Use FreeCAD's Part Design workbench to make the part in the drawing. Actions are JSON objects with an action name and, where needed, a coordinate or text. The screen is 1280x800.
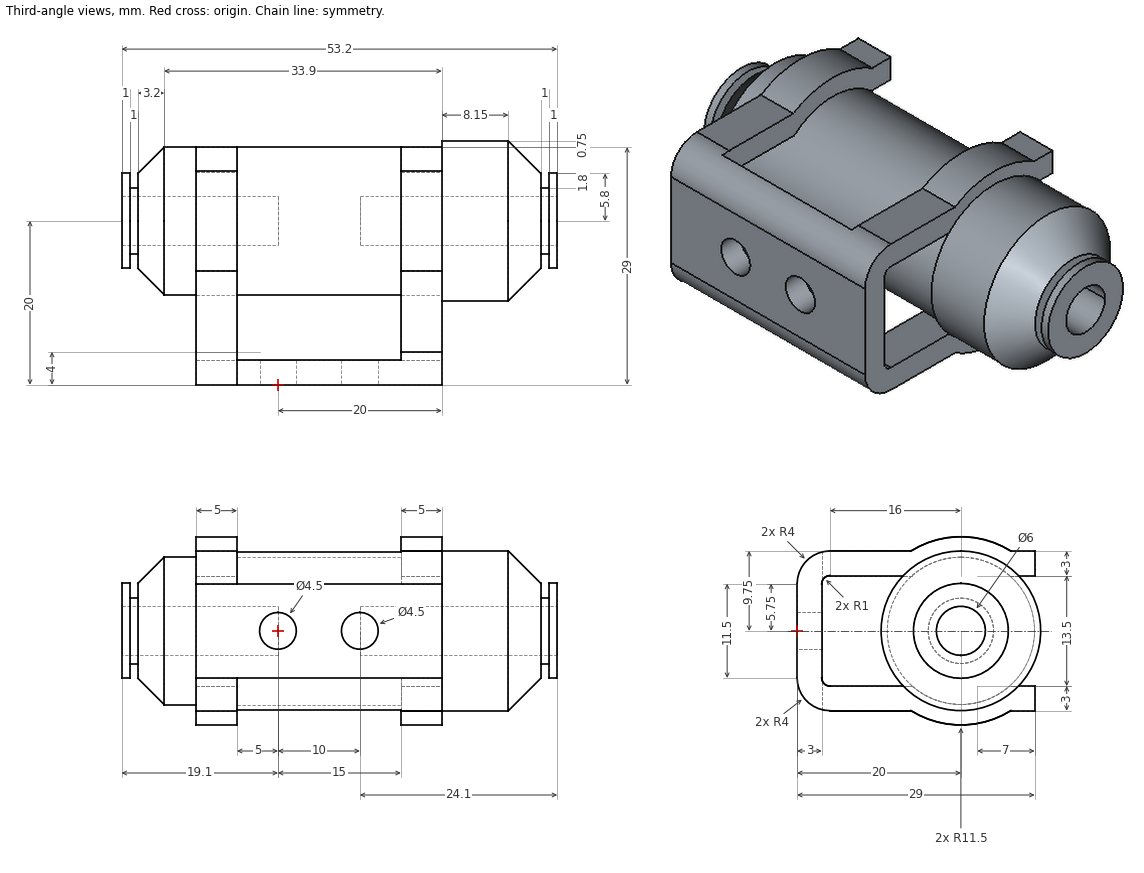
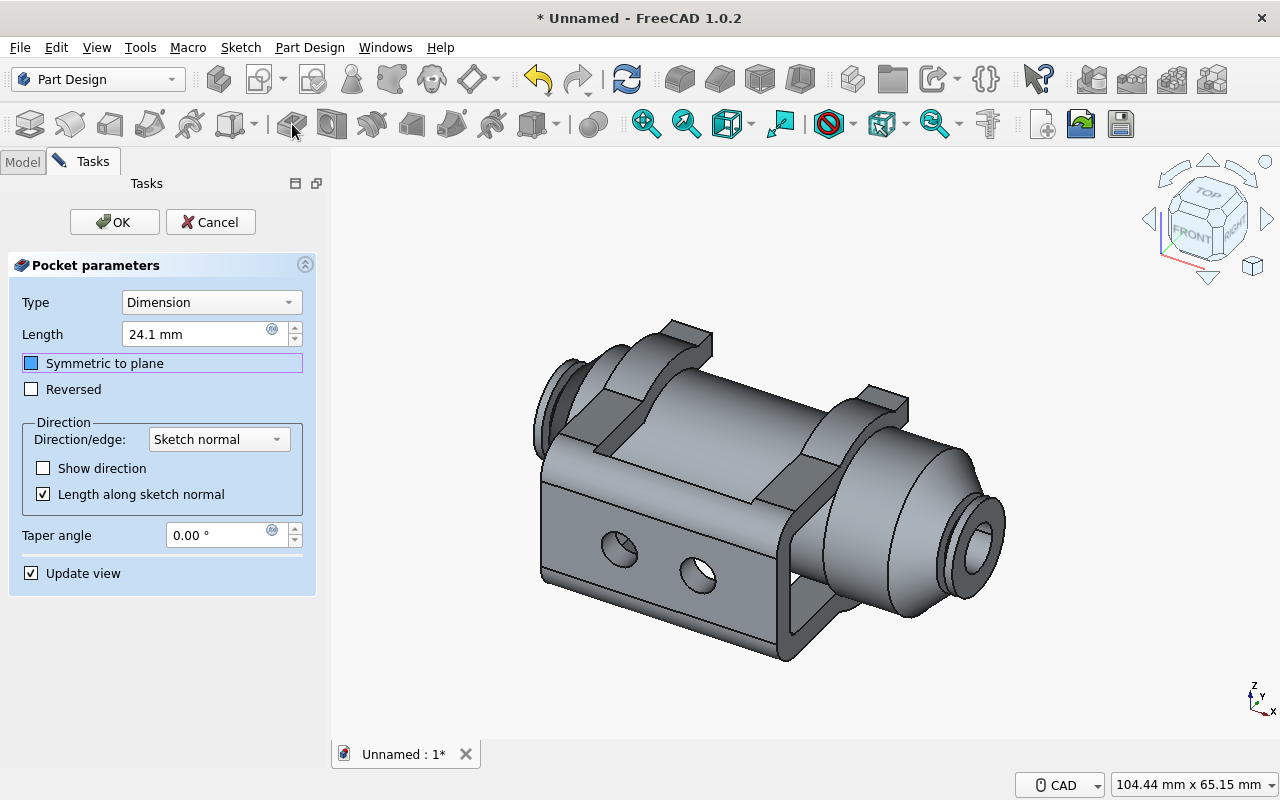
{"action": "left_click", "coordinate": [115, 222]}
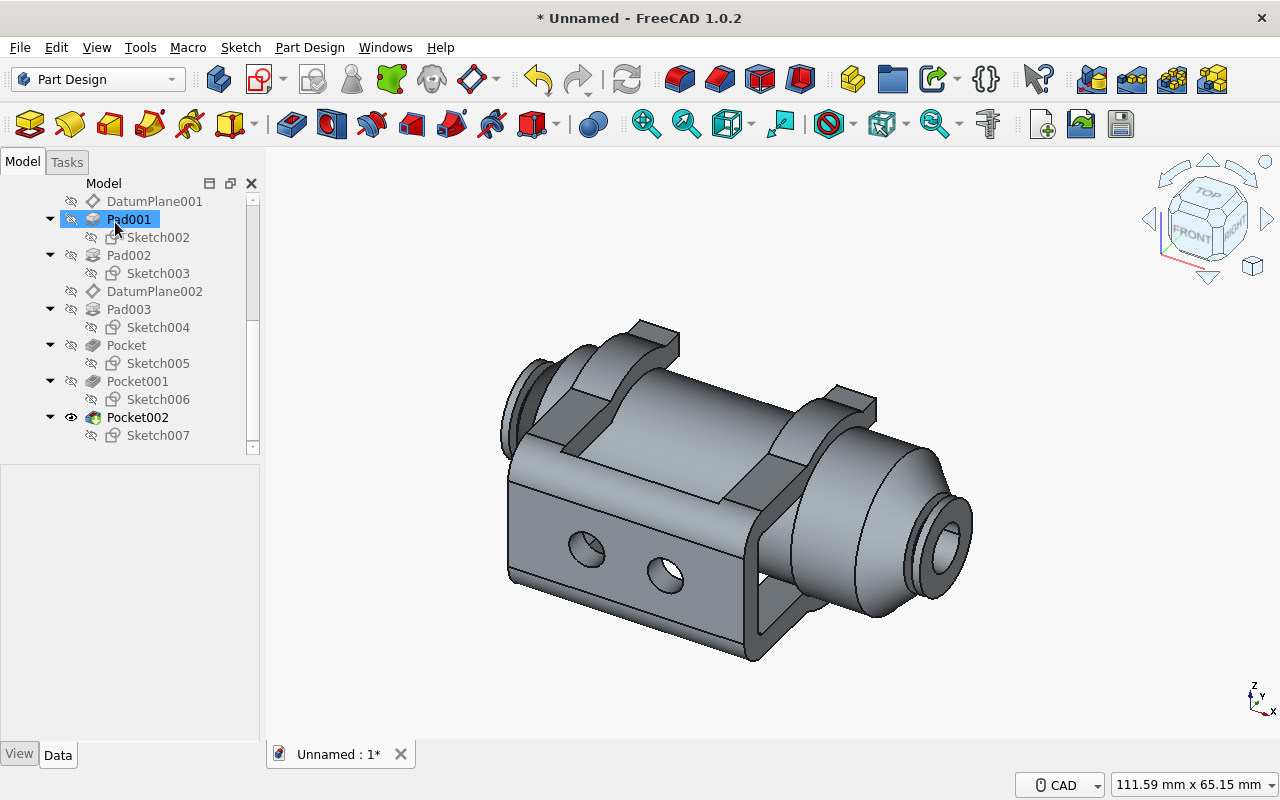
{"action": "left_click", "coordinate": [260, 80]}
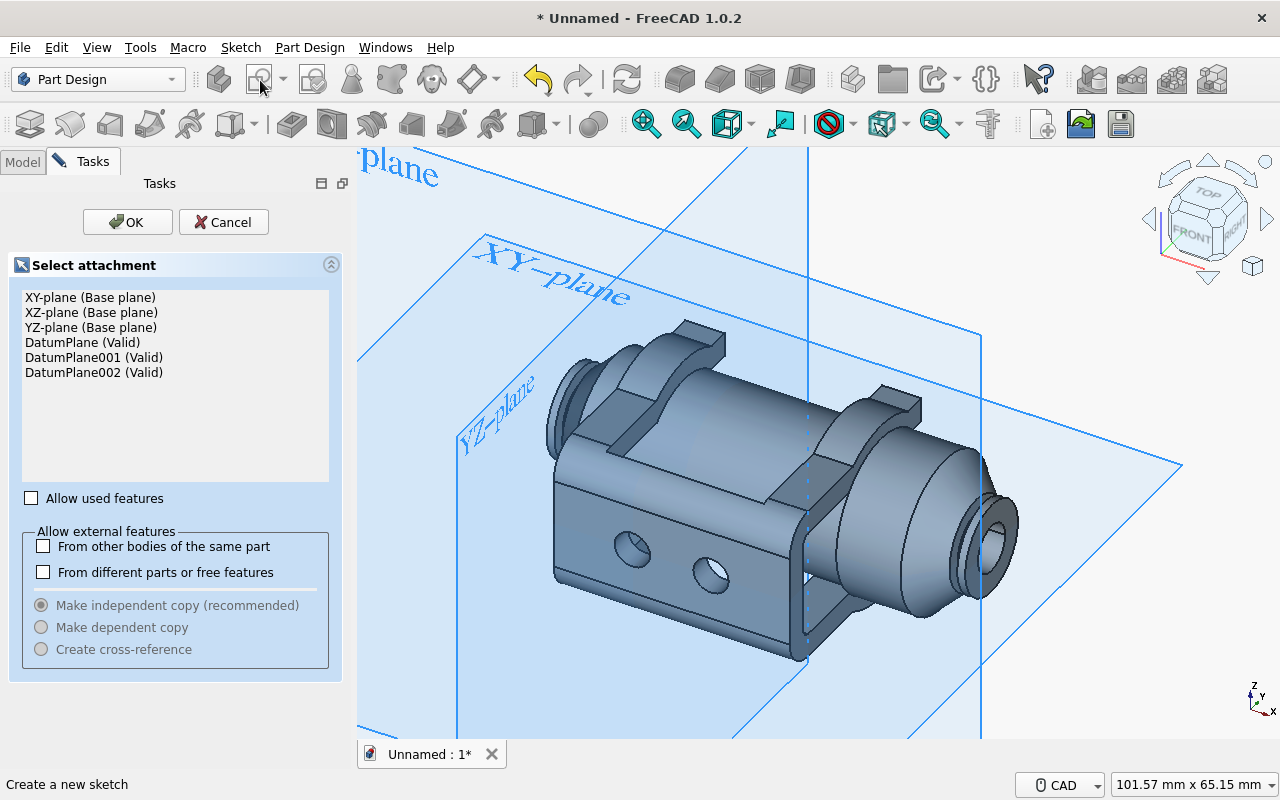
{"action": "left_click", "coordinate": [82, 328]}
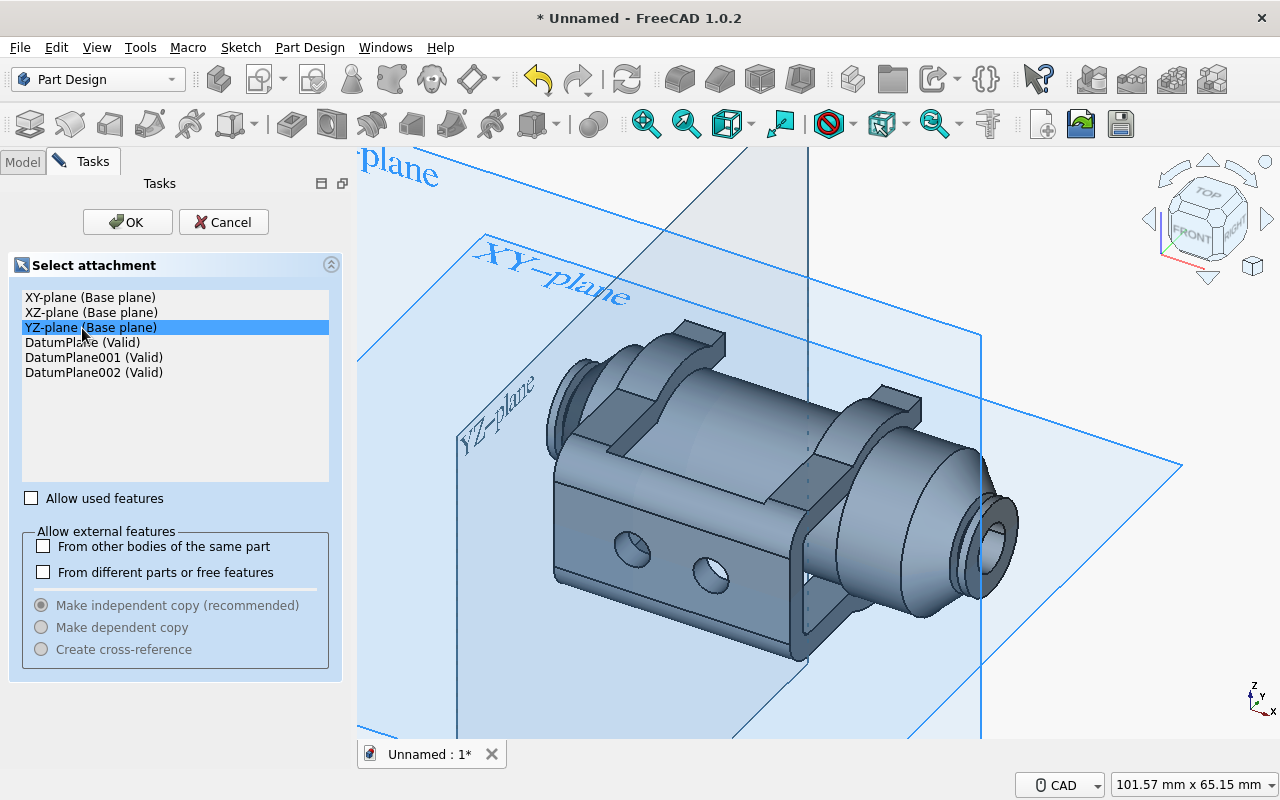
{"action": "left_click", "coordinate": [128, 222]}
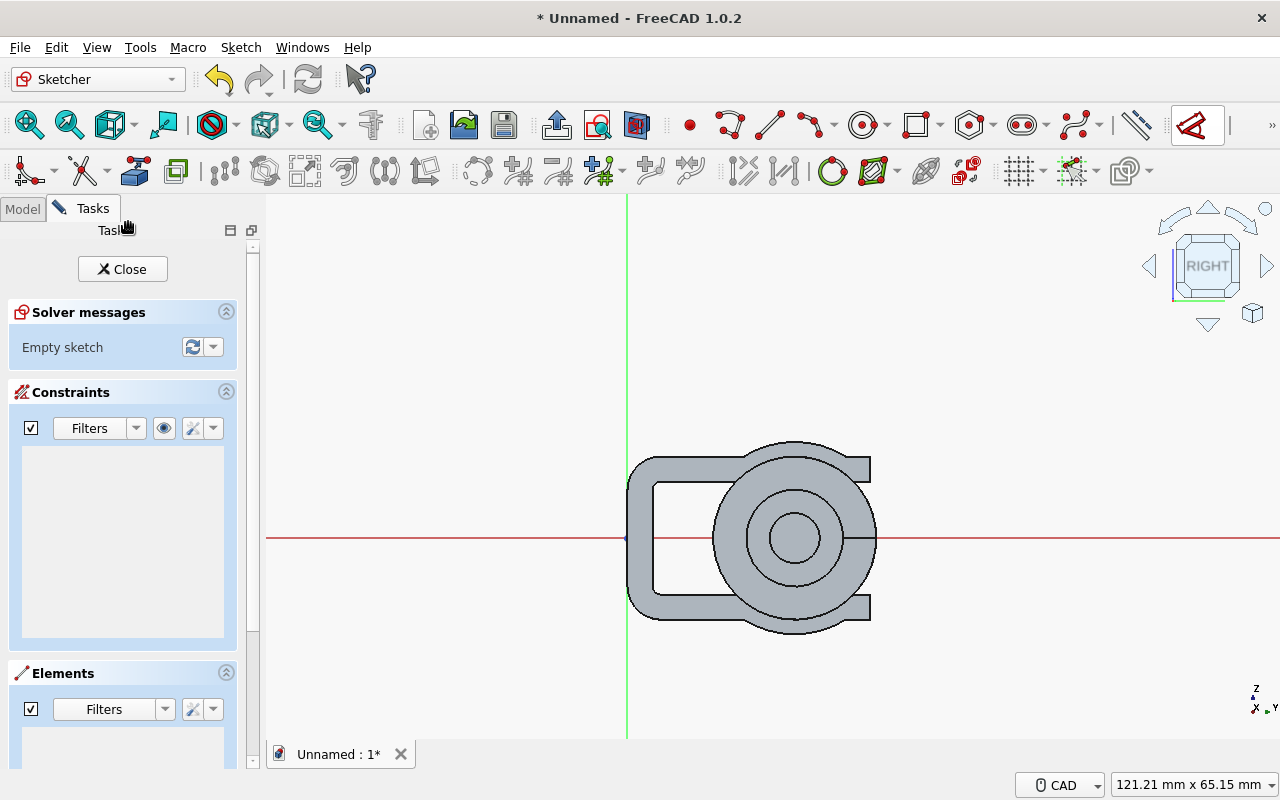
{"action": "left_click", "coordinate": [638, 126]}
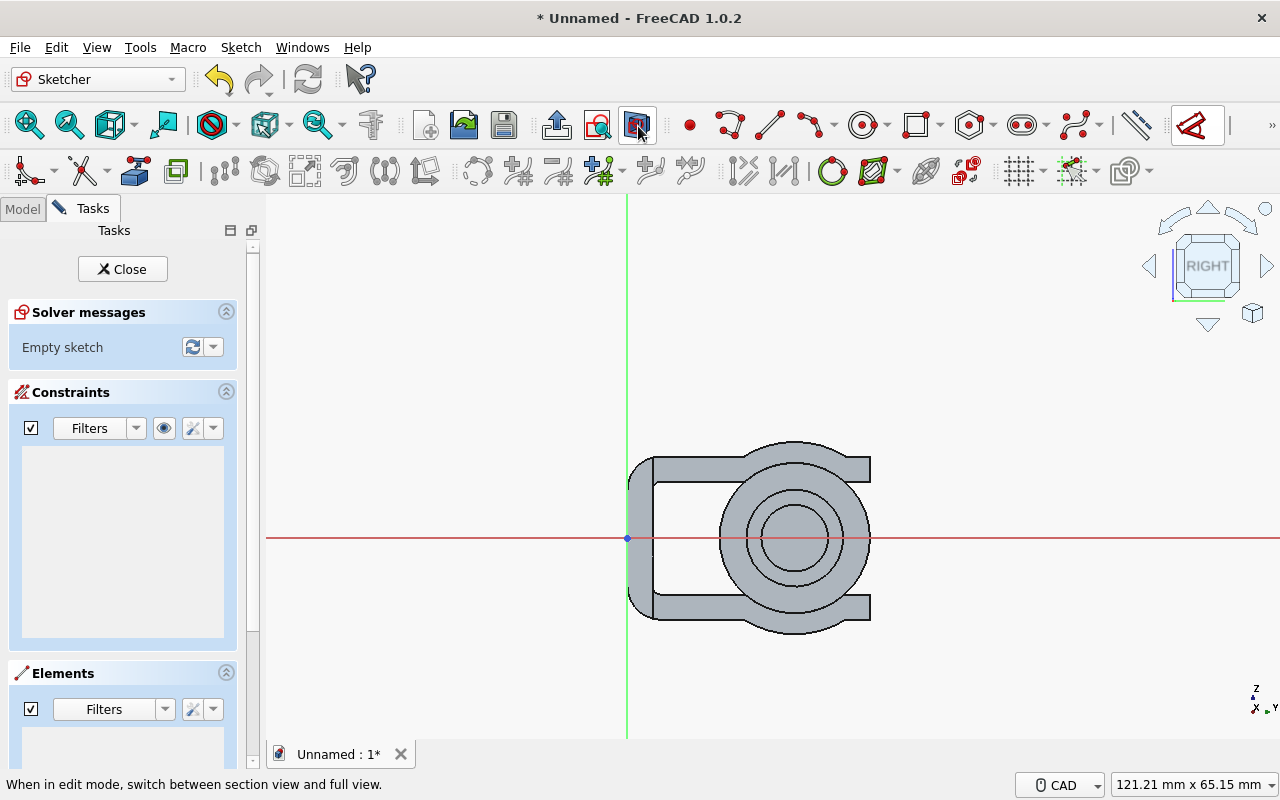
{"action": "scroll", "coordinate": [809, 549], "scroll_direction": "up", "scroll_amount": 10}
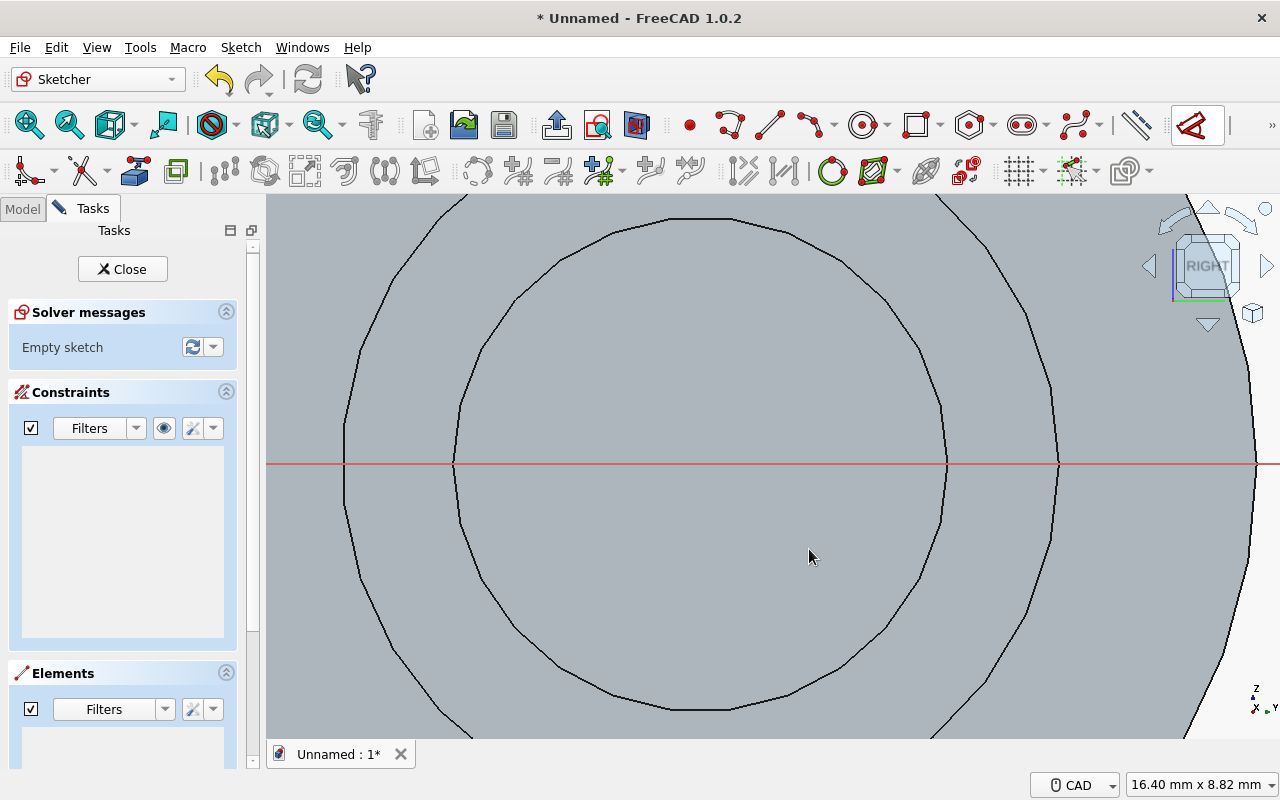
{"action": "left_click", "coordinate": [864, 126]}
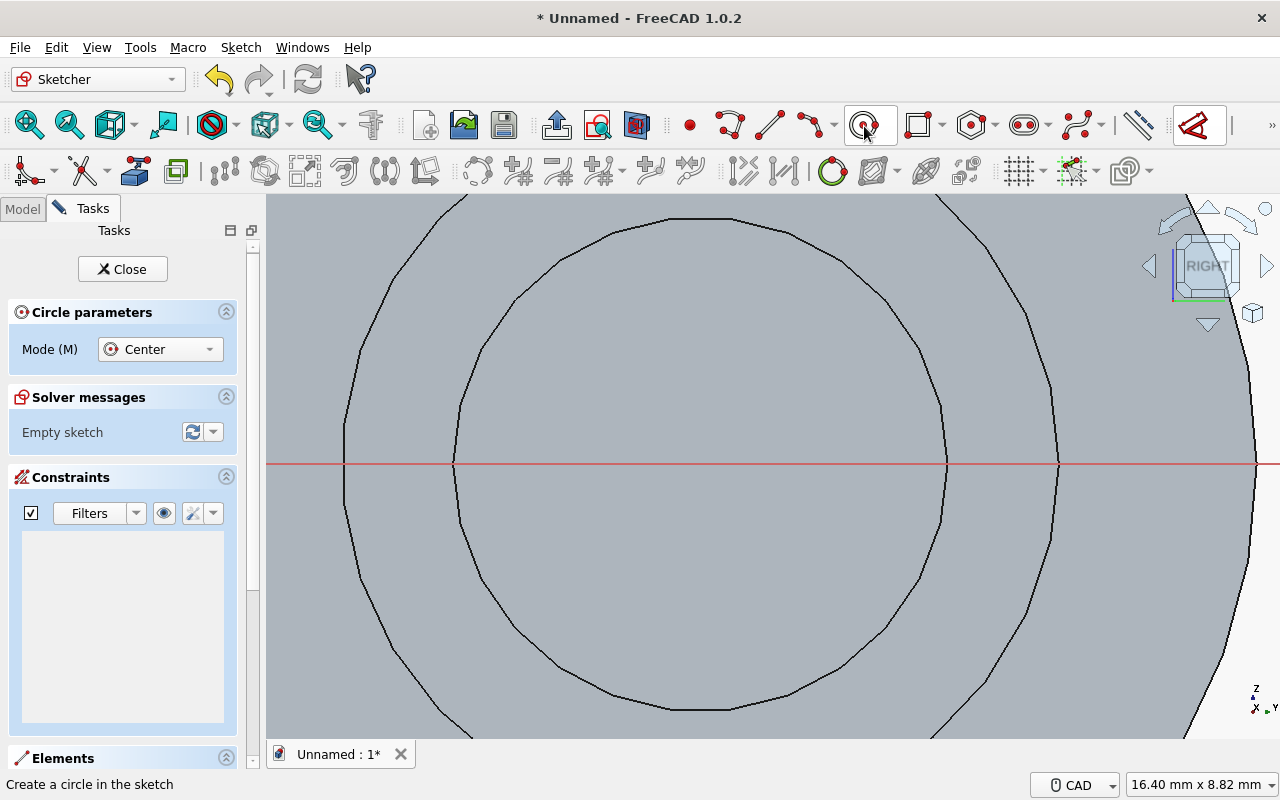
{"action": "left_click", "coordinate": [700, 464]}
{"action": "left_click", "coordinate": [831, 333]}
{"action": "key", "text": "Escape"}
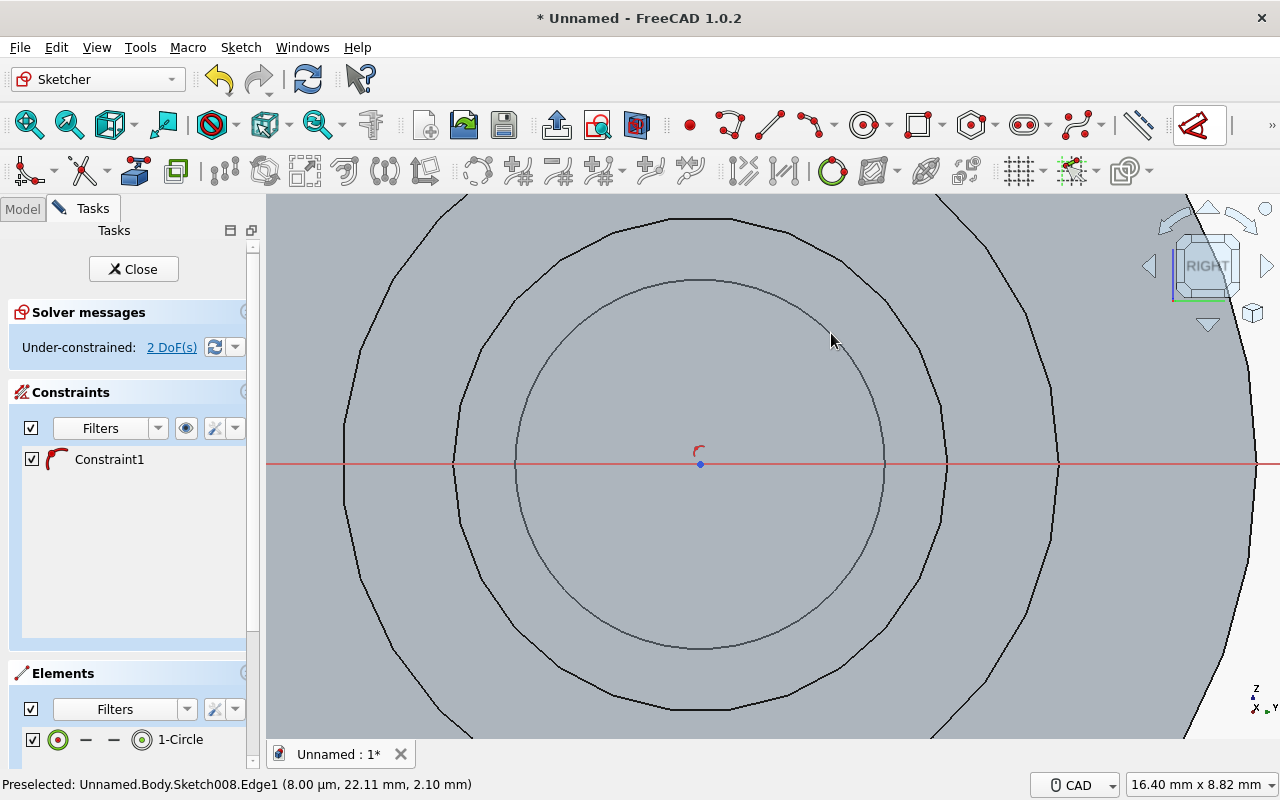
{"action": "left_click", "coordinate": [830, 333]}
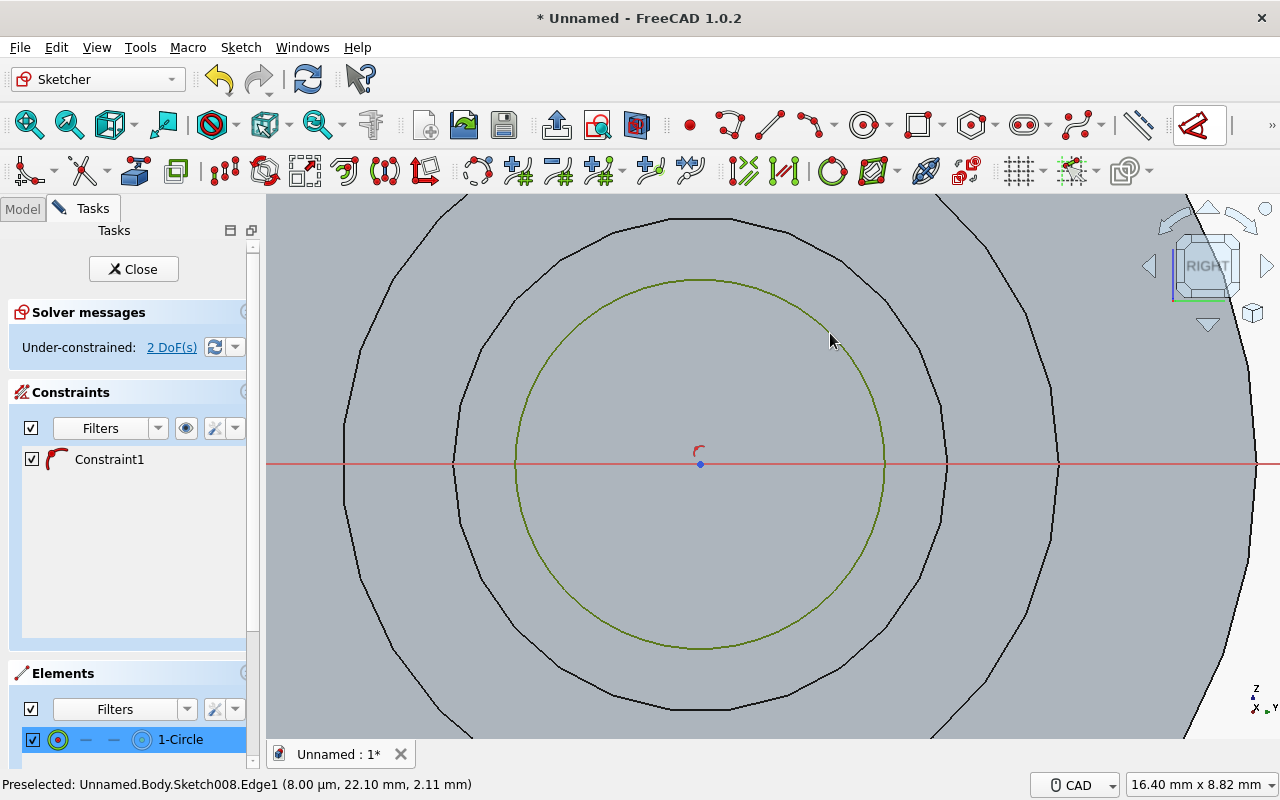
{"action": "left_click", "coordinate": [1220, 126]}